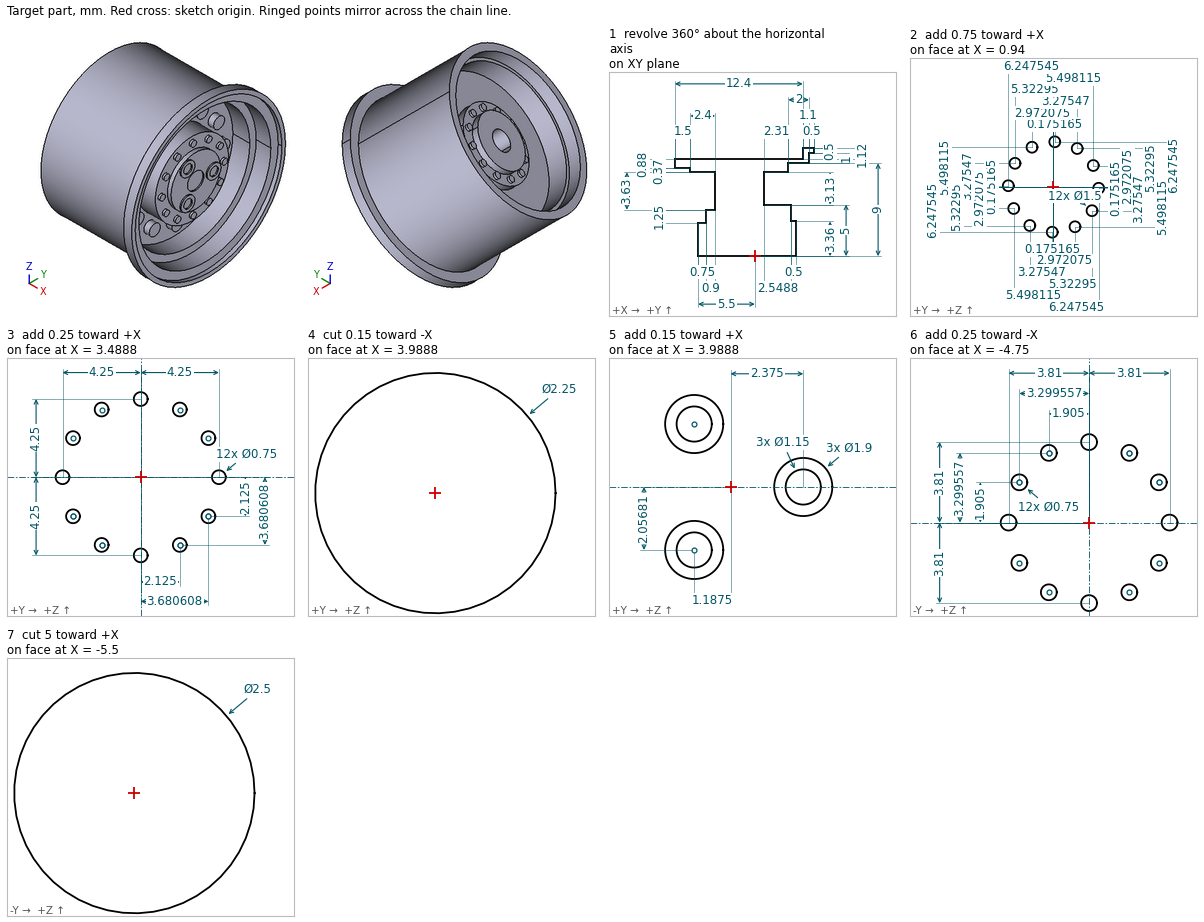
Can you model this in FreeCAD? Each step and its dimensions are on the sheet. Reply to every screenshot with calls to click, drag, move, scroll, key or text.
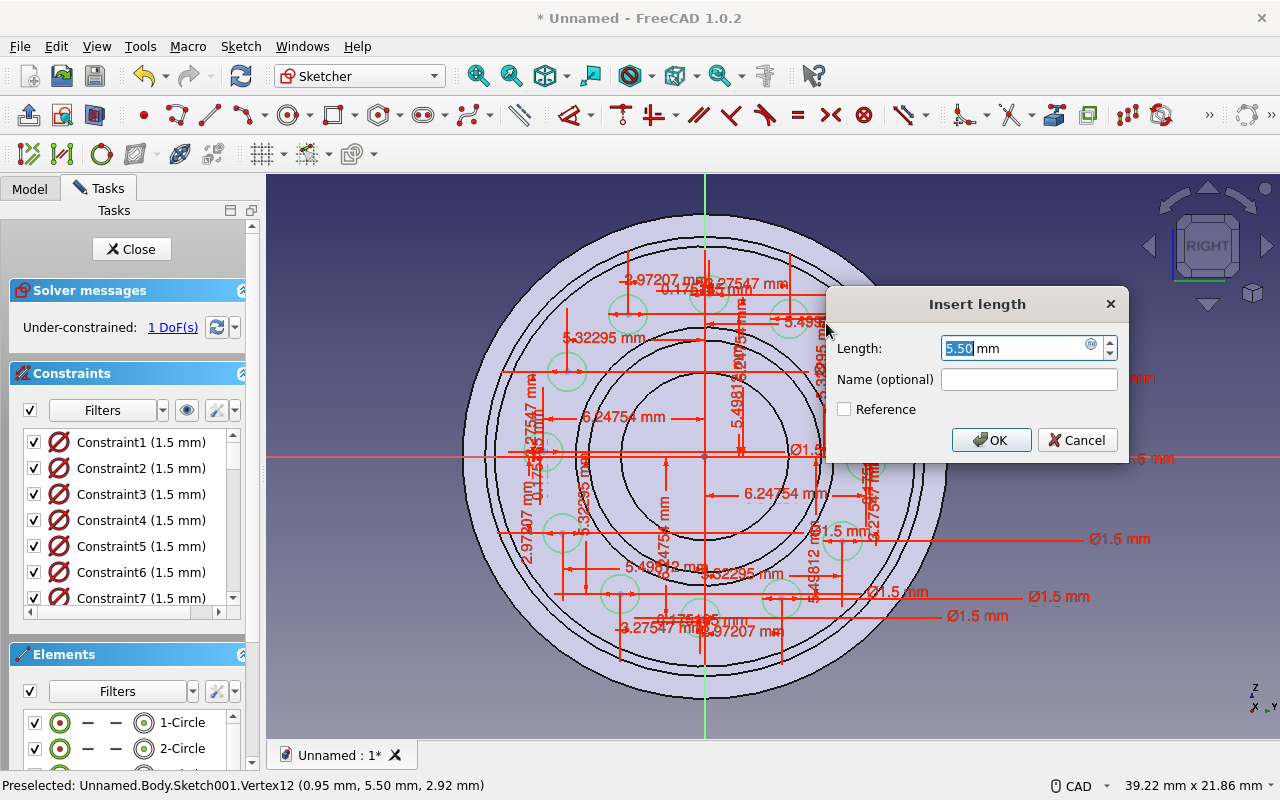
text(5.498115)
key(Return)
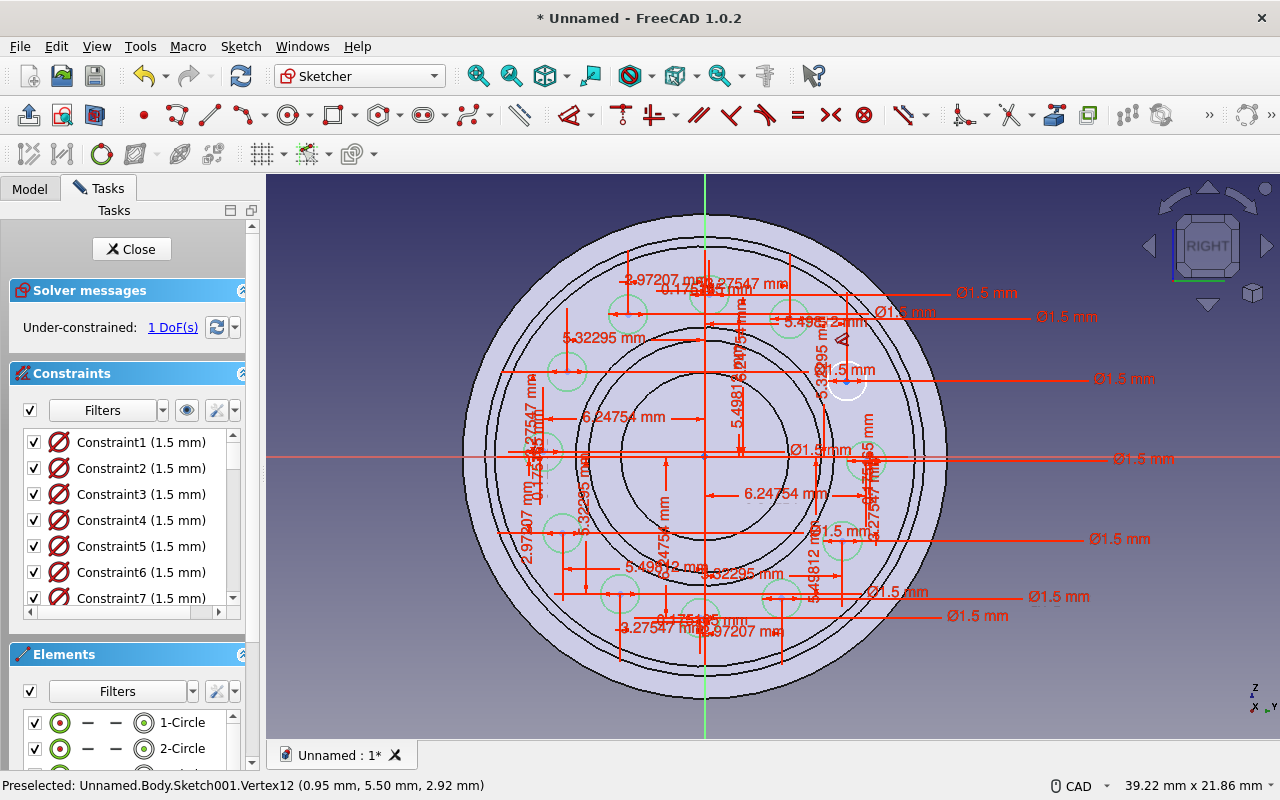
click(847, 381)
click(881, 419)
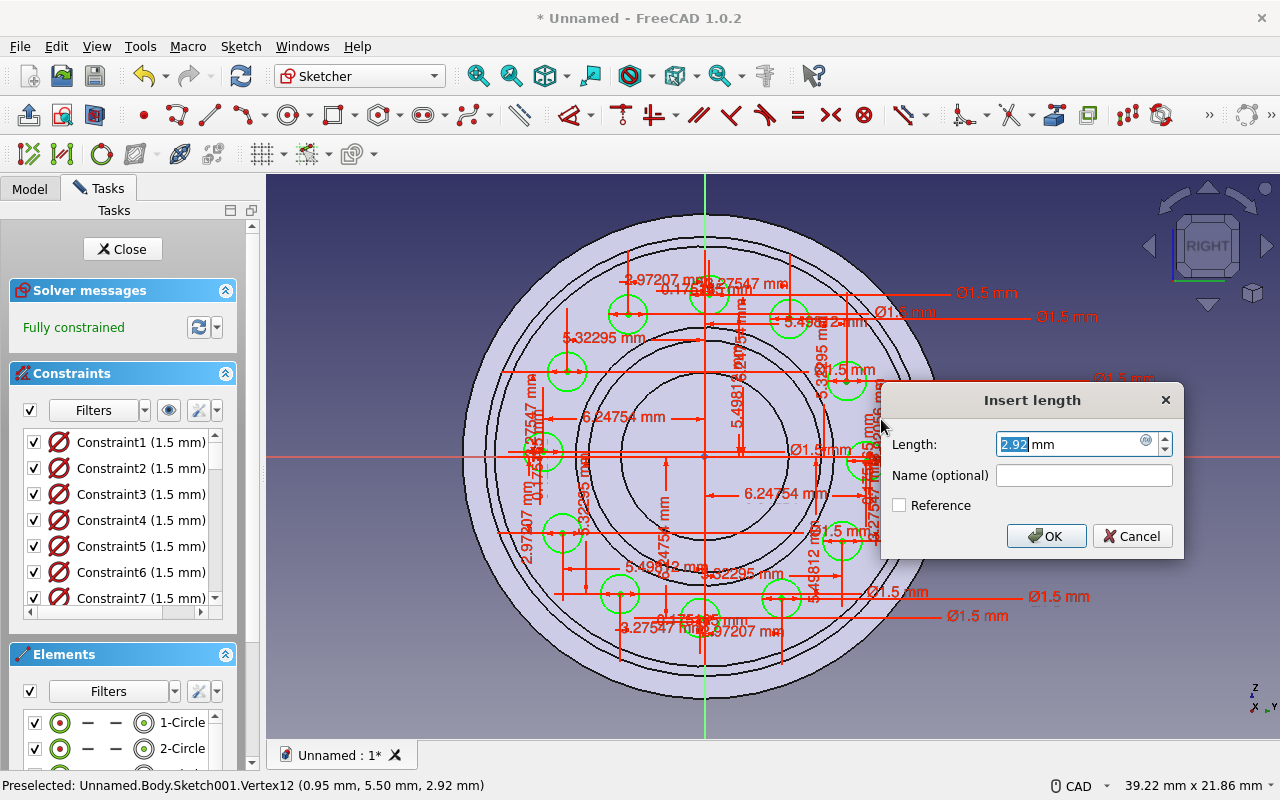
text(2.972075)
key(Return)
key(Escape)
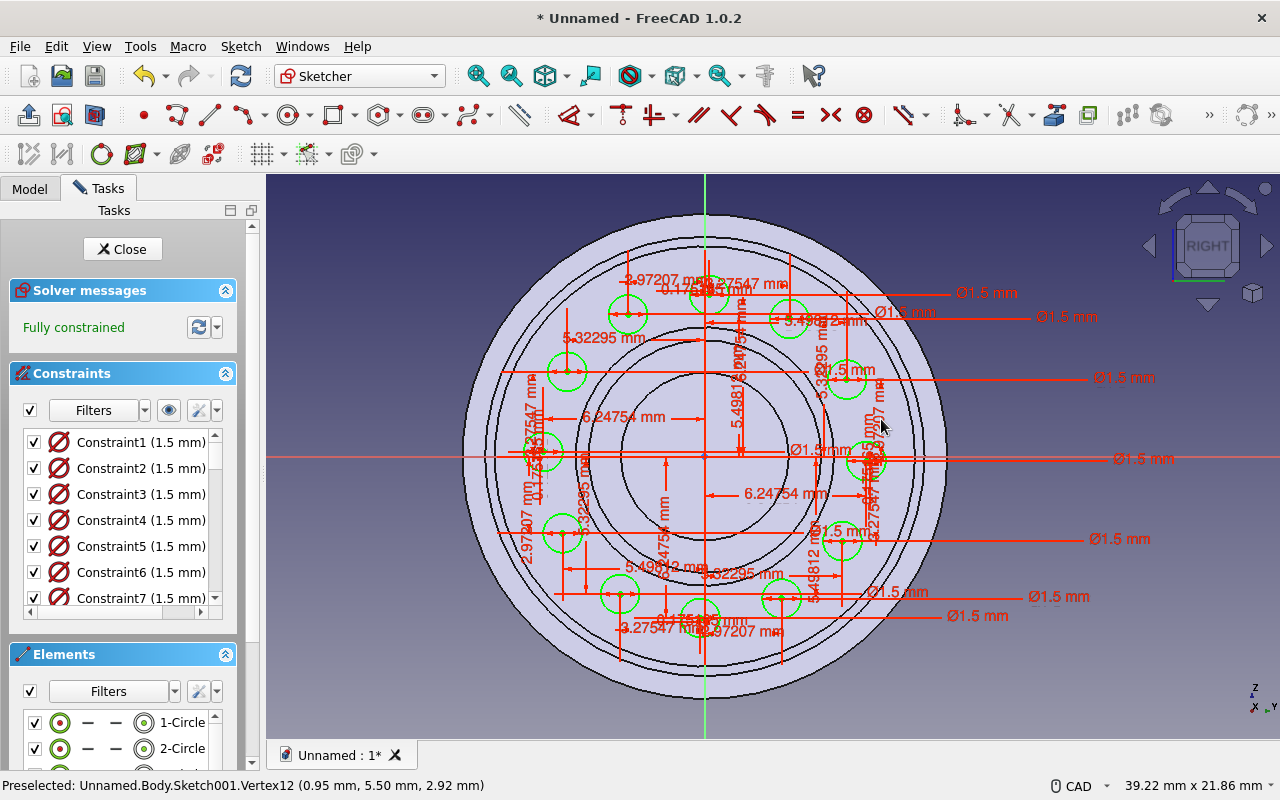
click(123, 249)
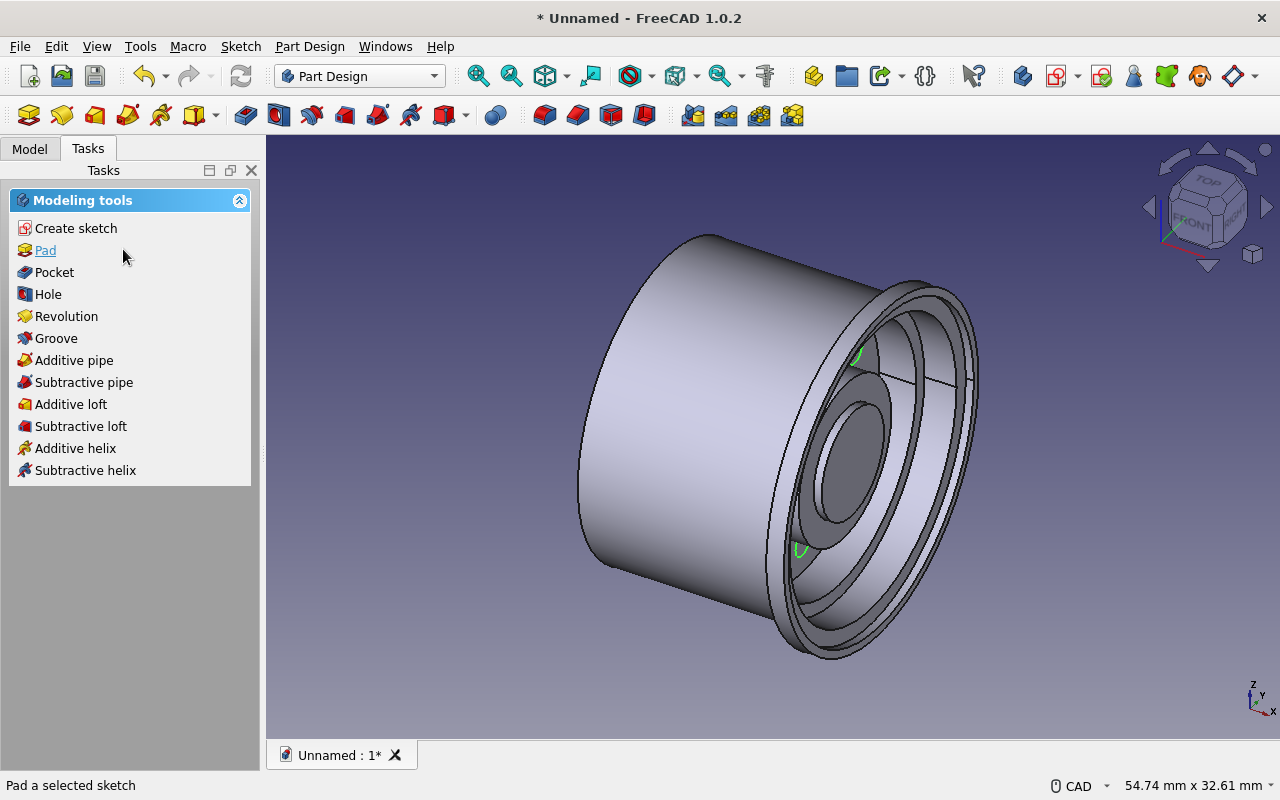
click(29, 116)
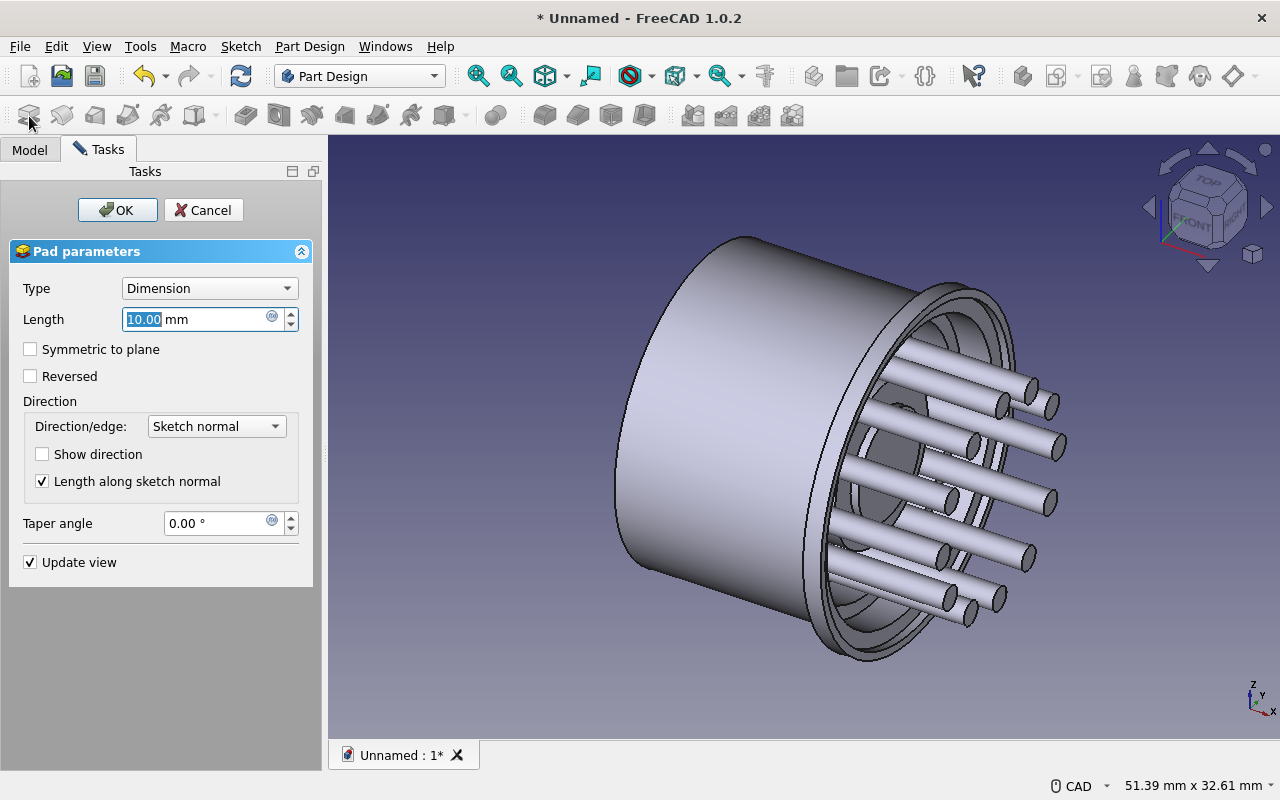
text(0.75)
key(Tab)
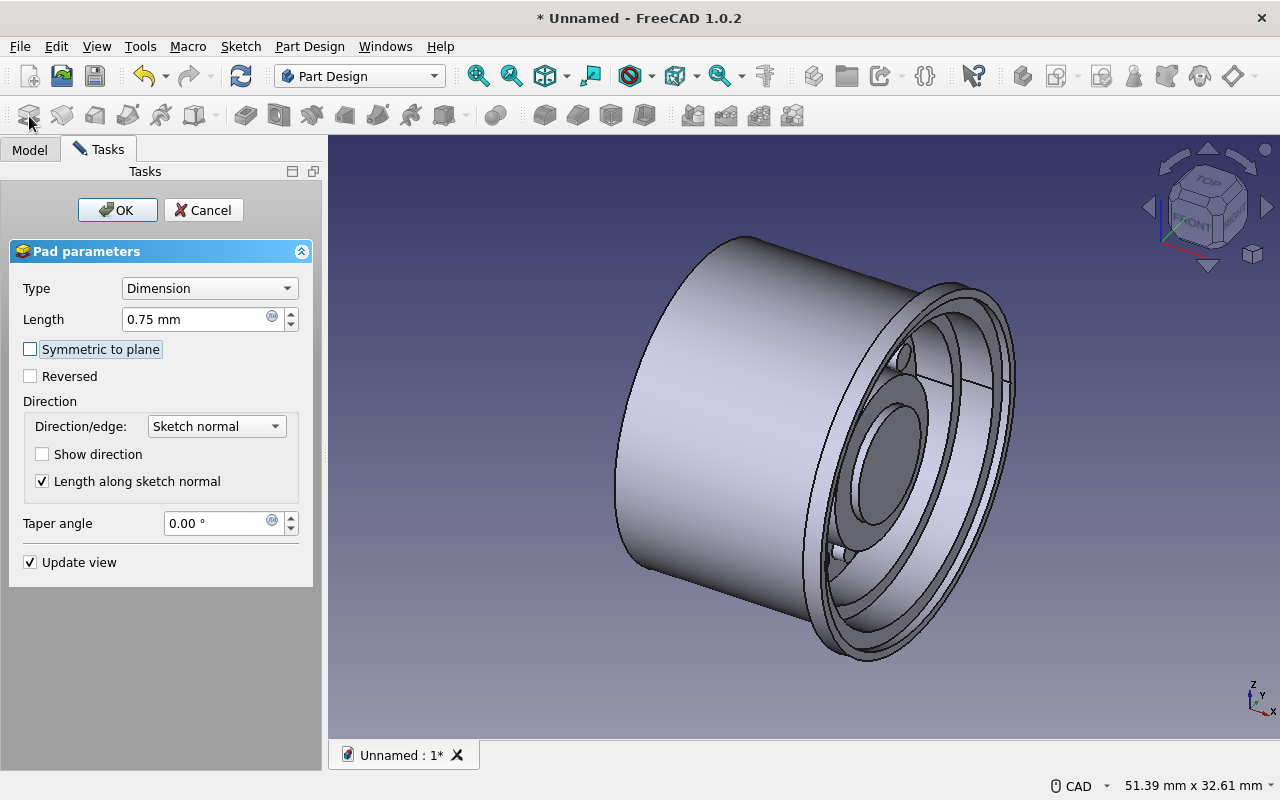
click(118, 210)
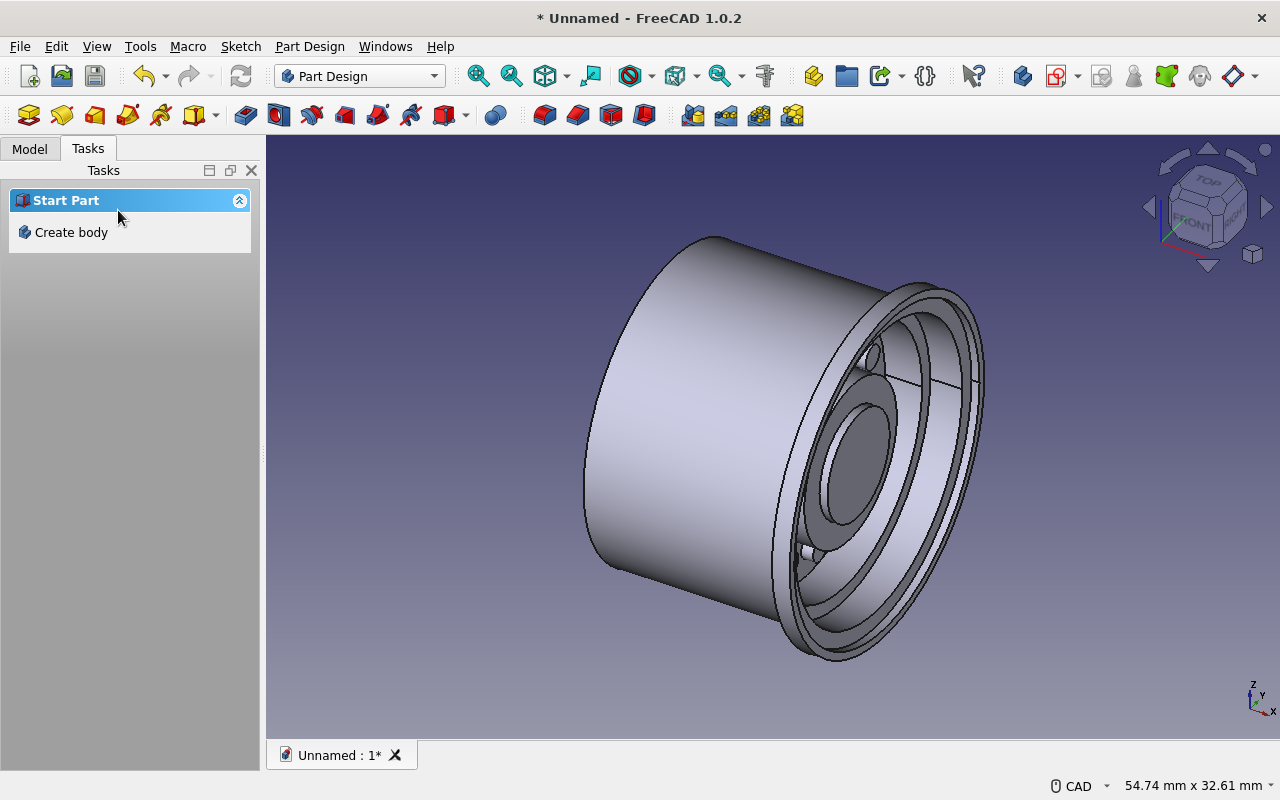
click(877, 392)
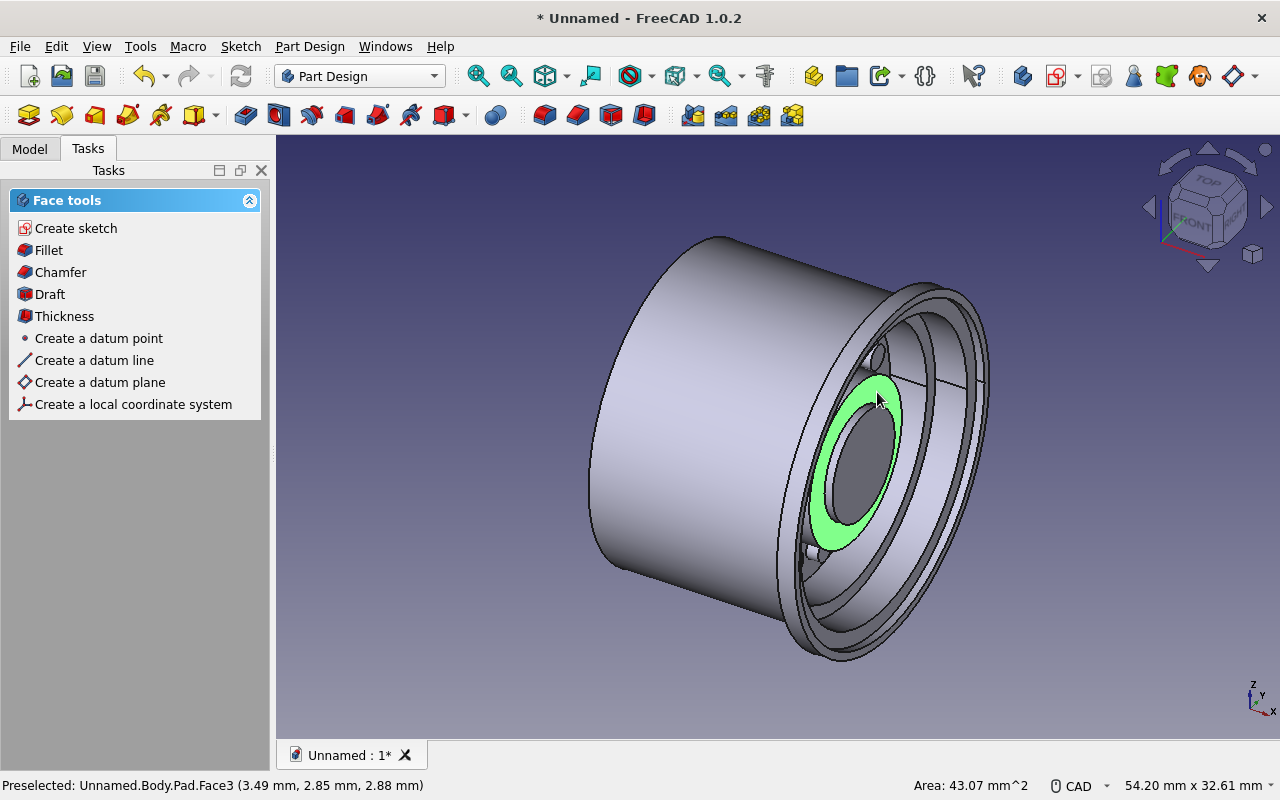
click(1056, 76)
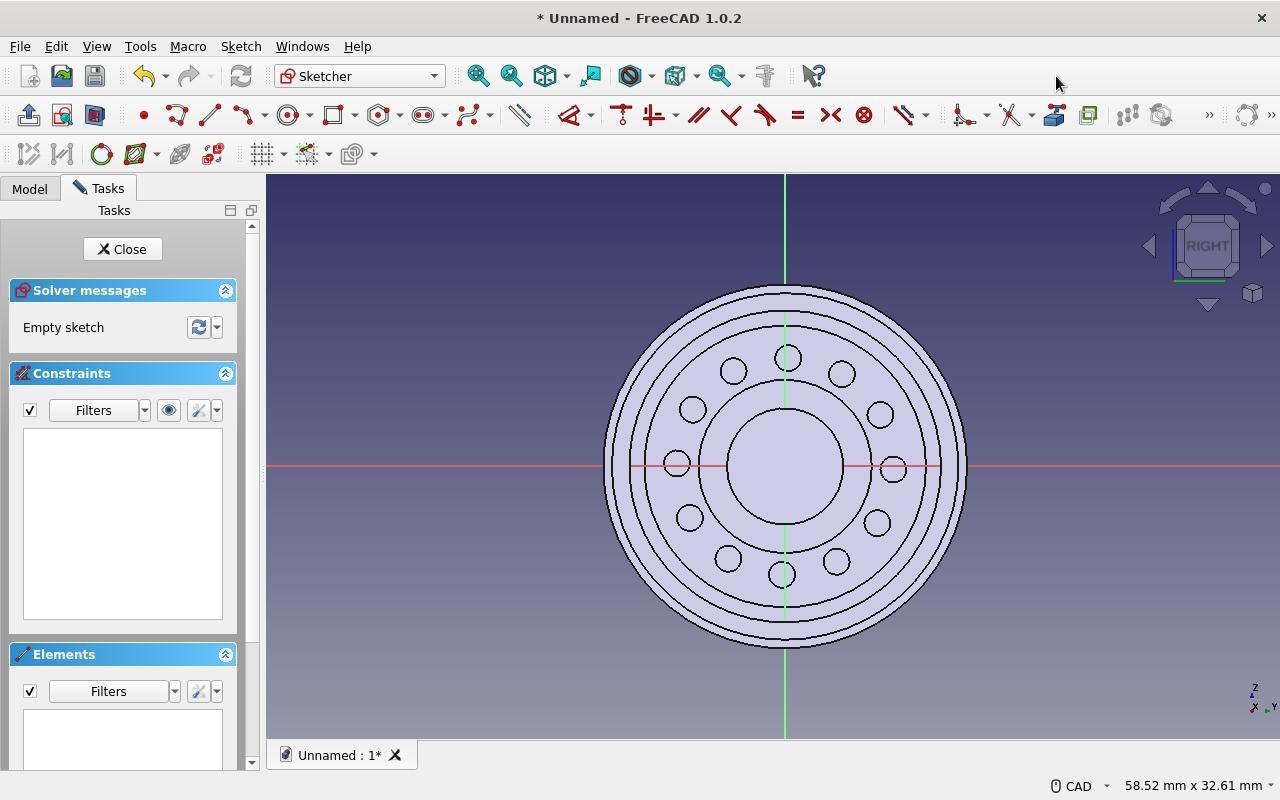
scroll(851, 475, up, 4)